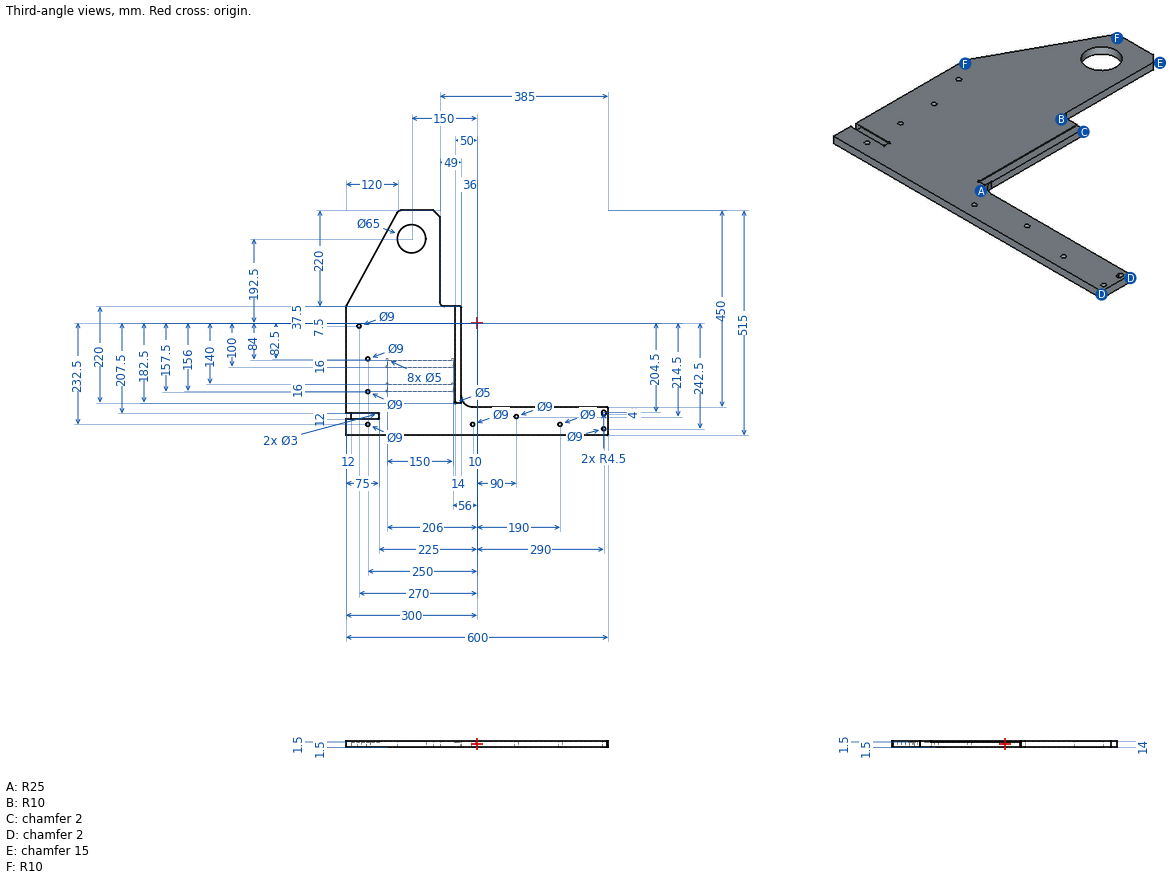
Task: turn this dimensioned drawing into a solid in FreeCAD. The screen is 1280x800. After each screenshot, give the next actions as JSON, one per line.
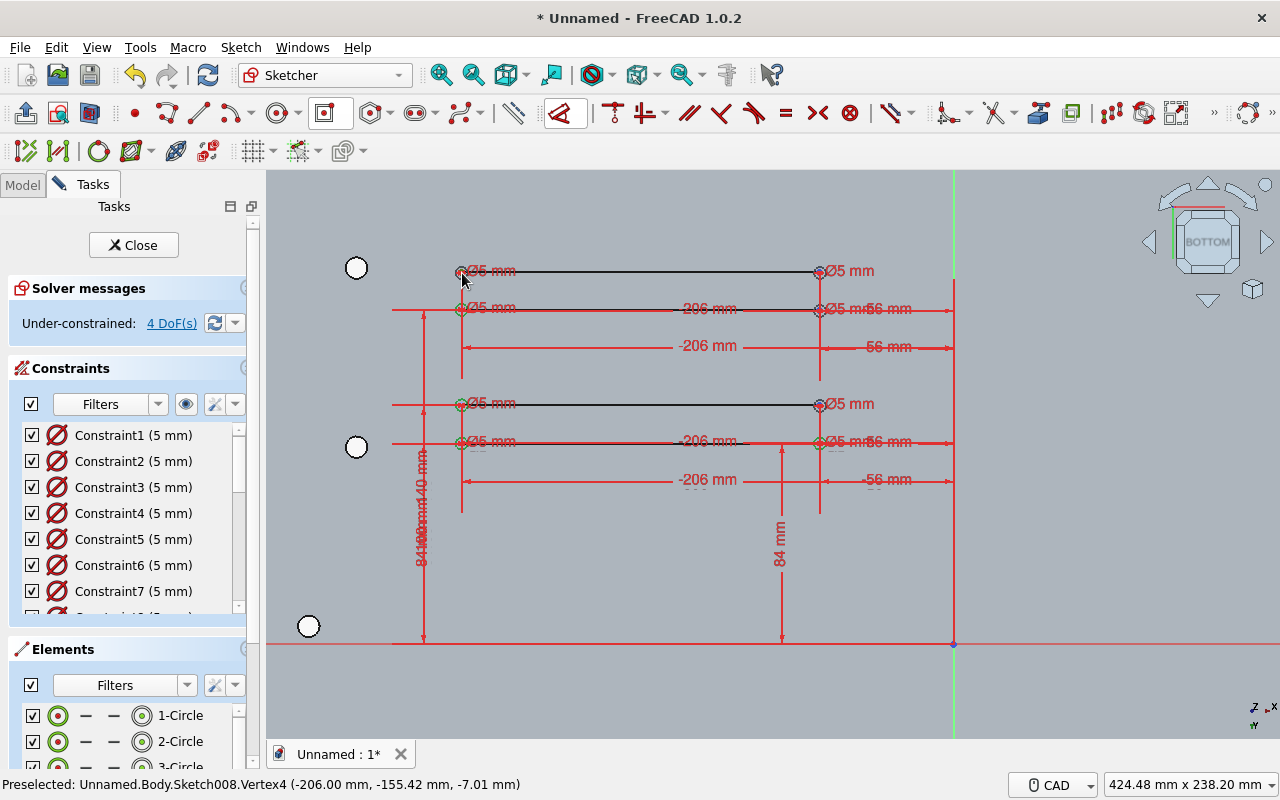
{"action": "left_click", "coordinate": [582, 114]}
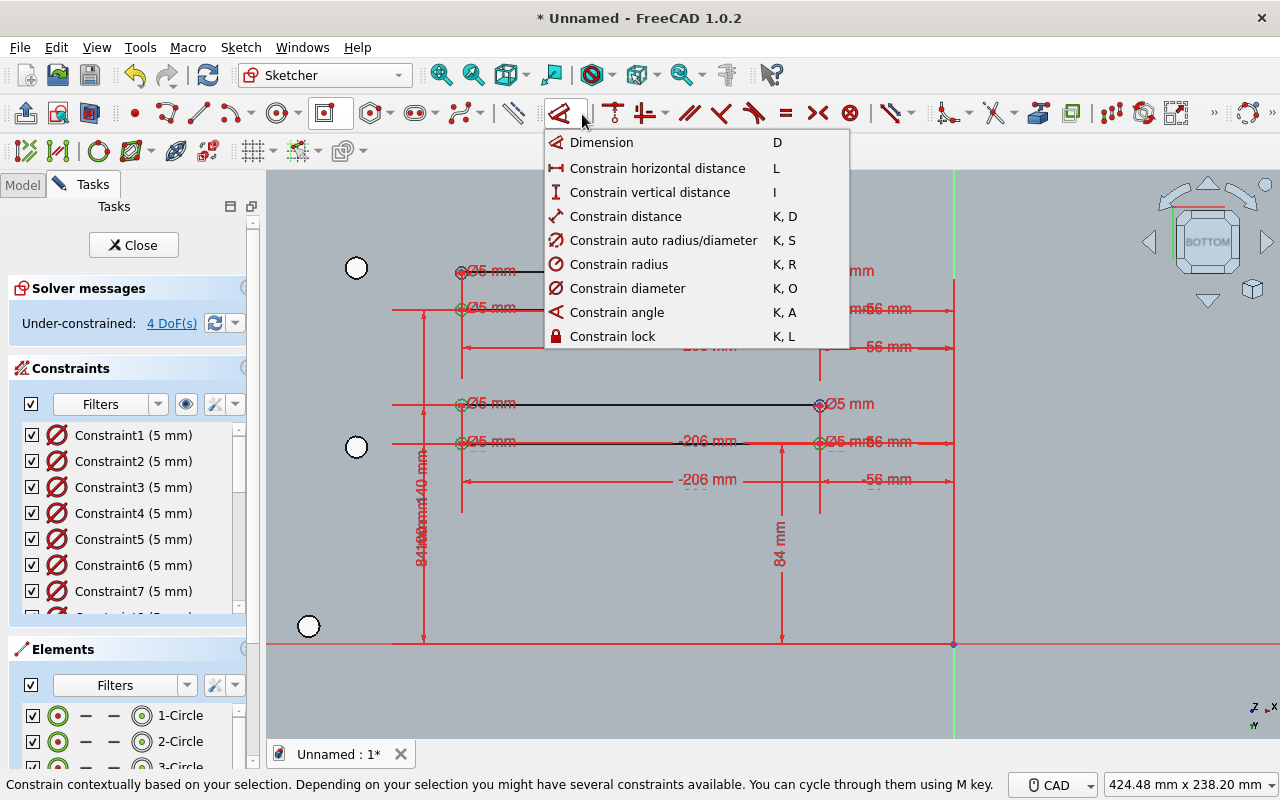
{"action": "left_click", "coordinate": [697, 192]}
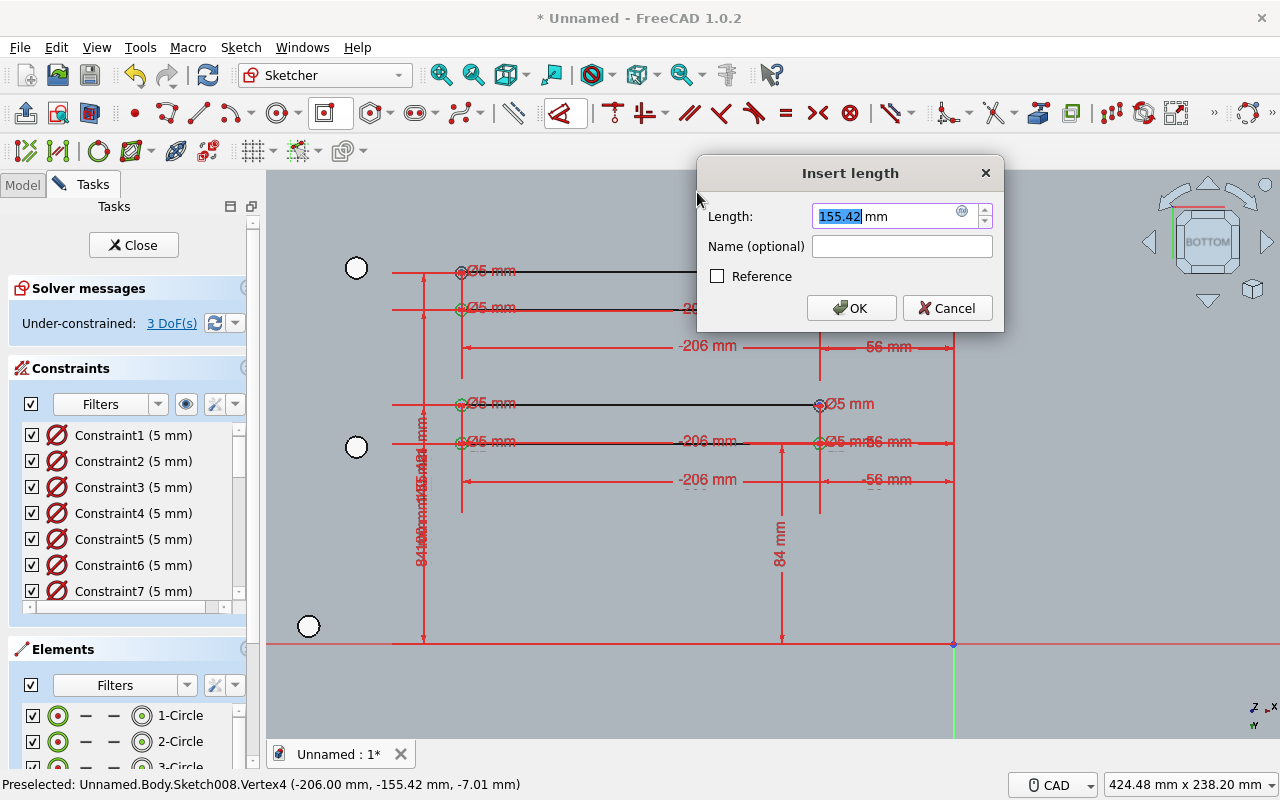
{"action": "type", "text": "156"}
{"action": "key", "text": "Return"}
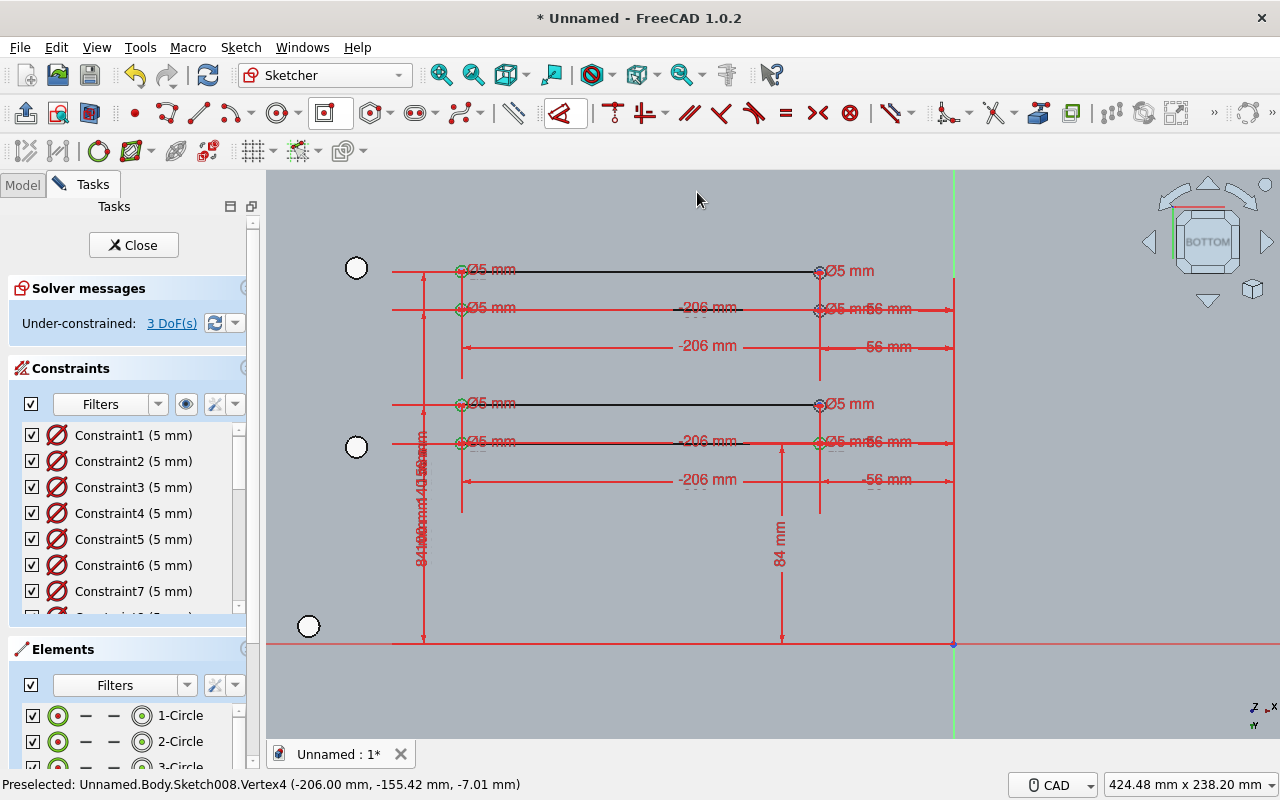
{"action": "left_click", "coordinate": [820, 406]}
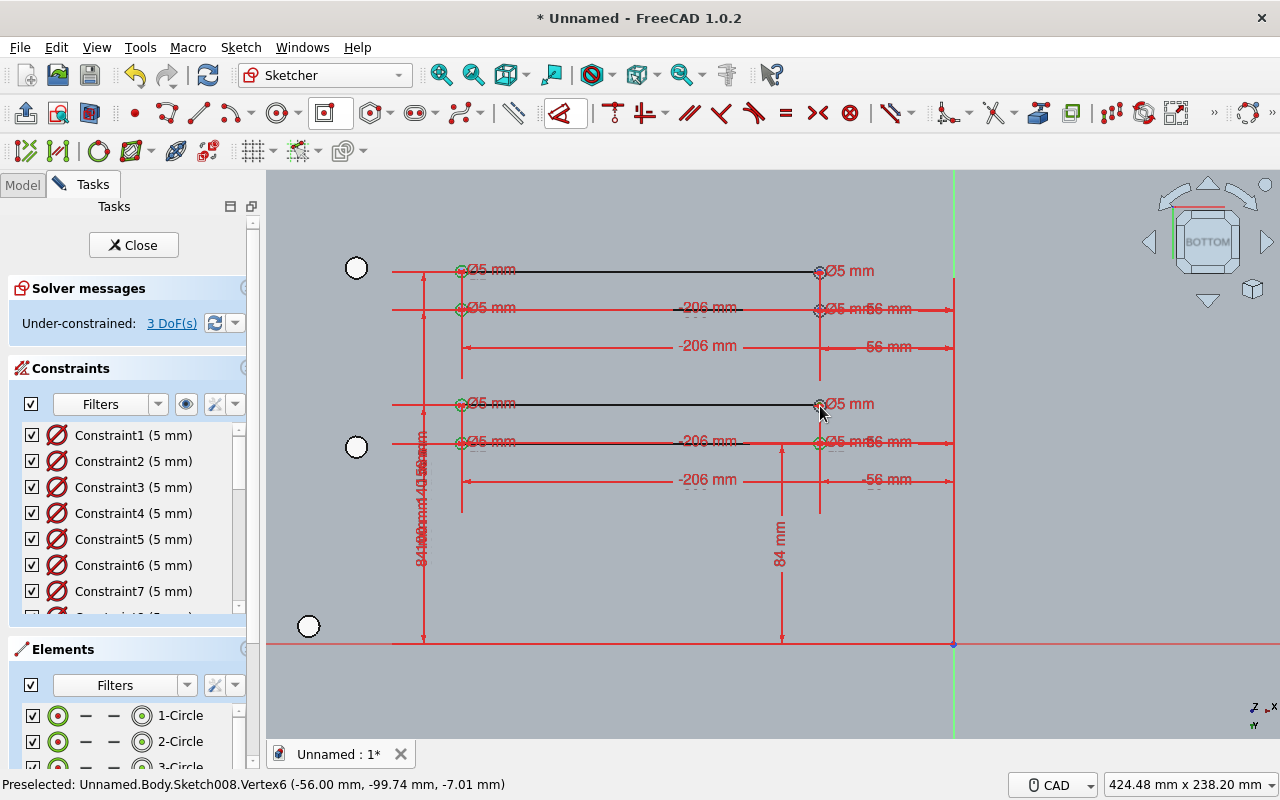
{"action": "key", "text": "i"}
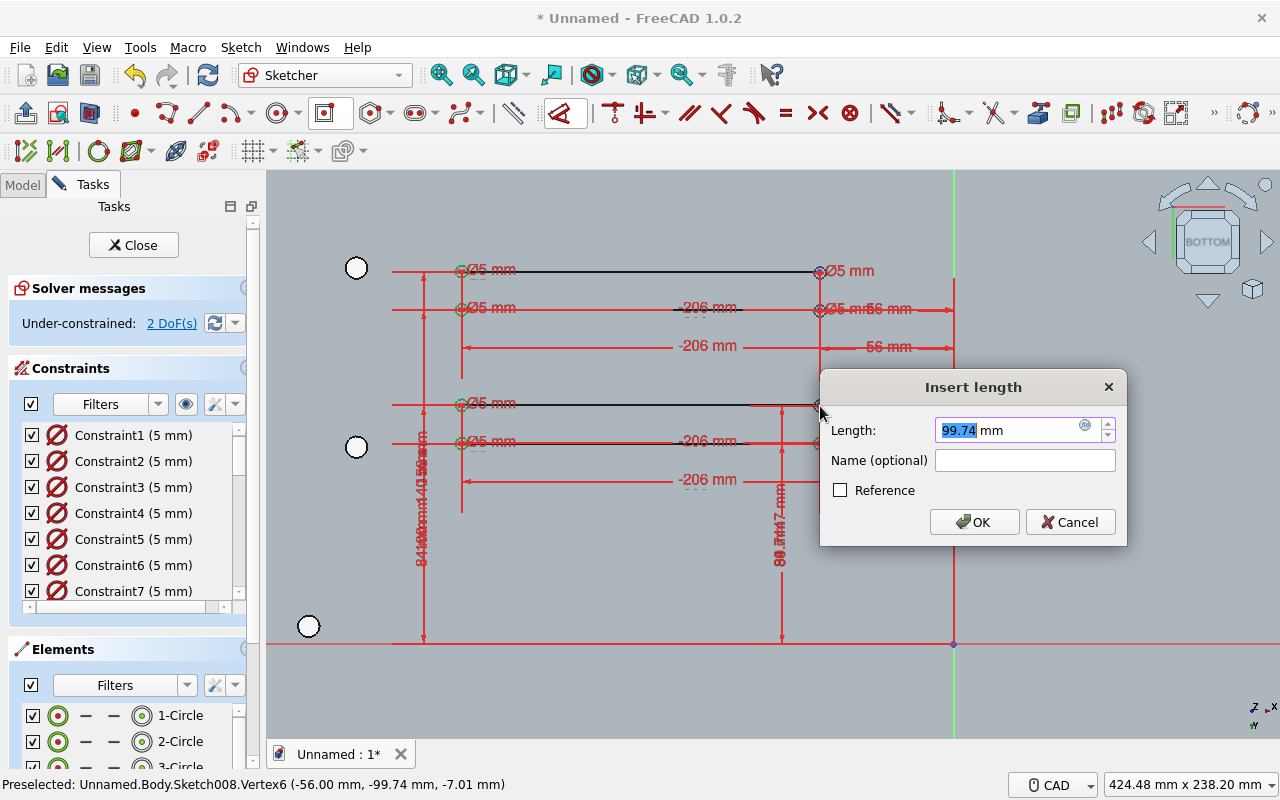
{"action": "type", "text": "100"}
{"action": "key", "text": "Return"}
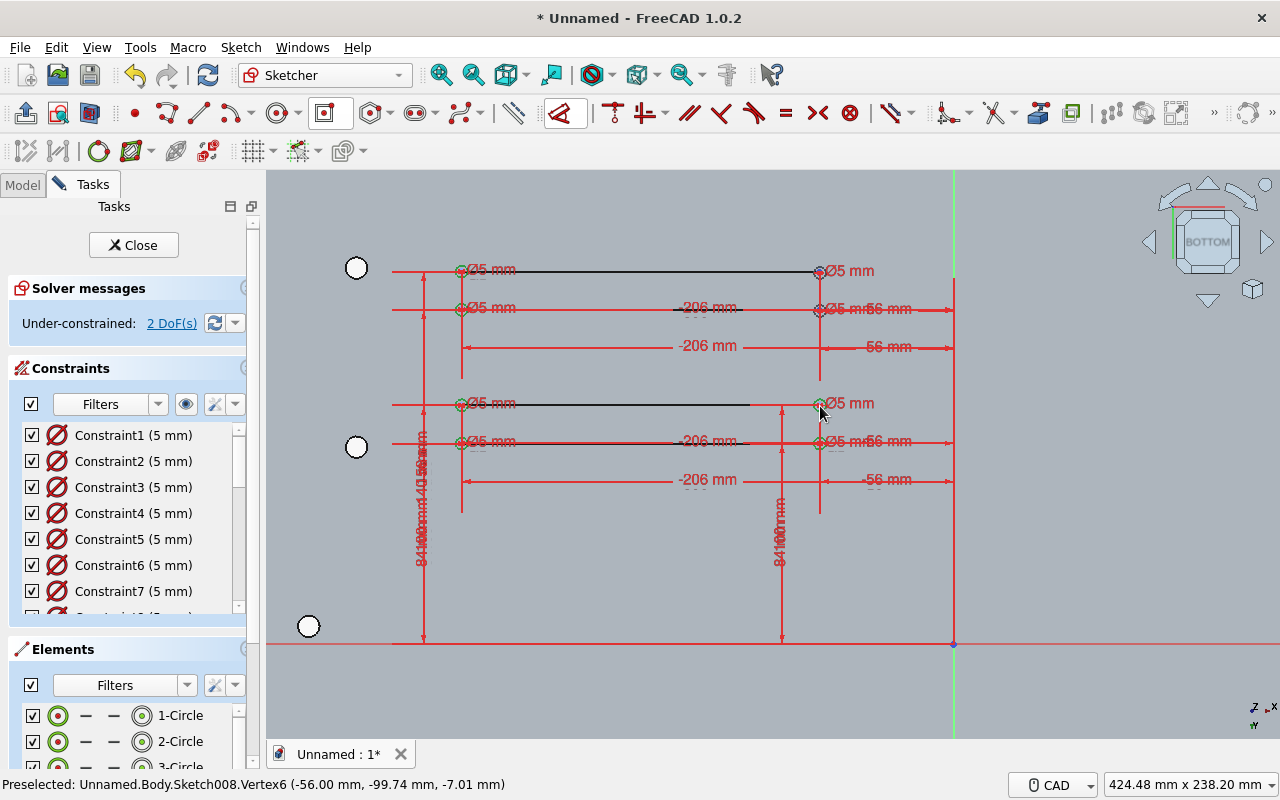
{"action": "left_click", "coordinate": [820, 311]}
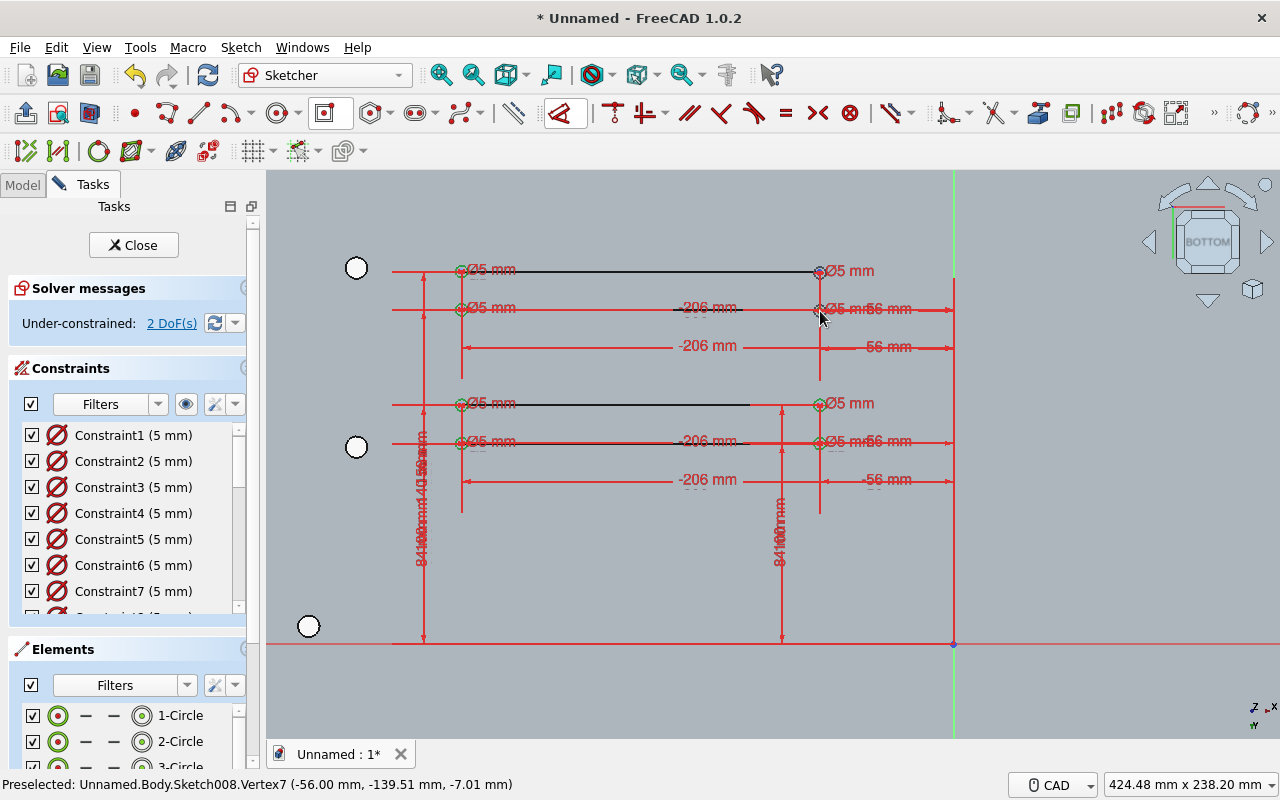
{"action": "left_click", "coordinate": [582, 114]}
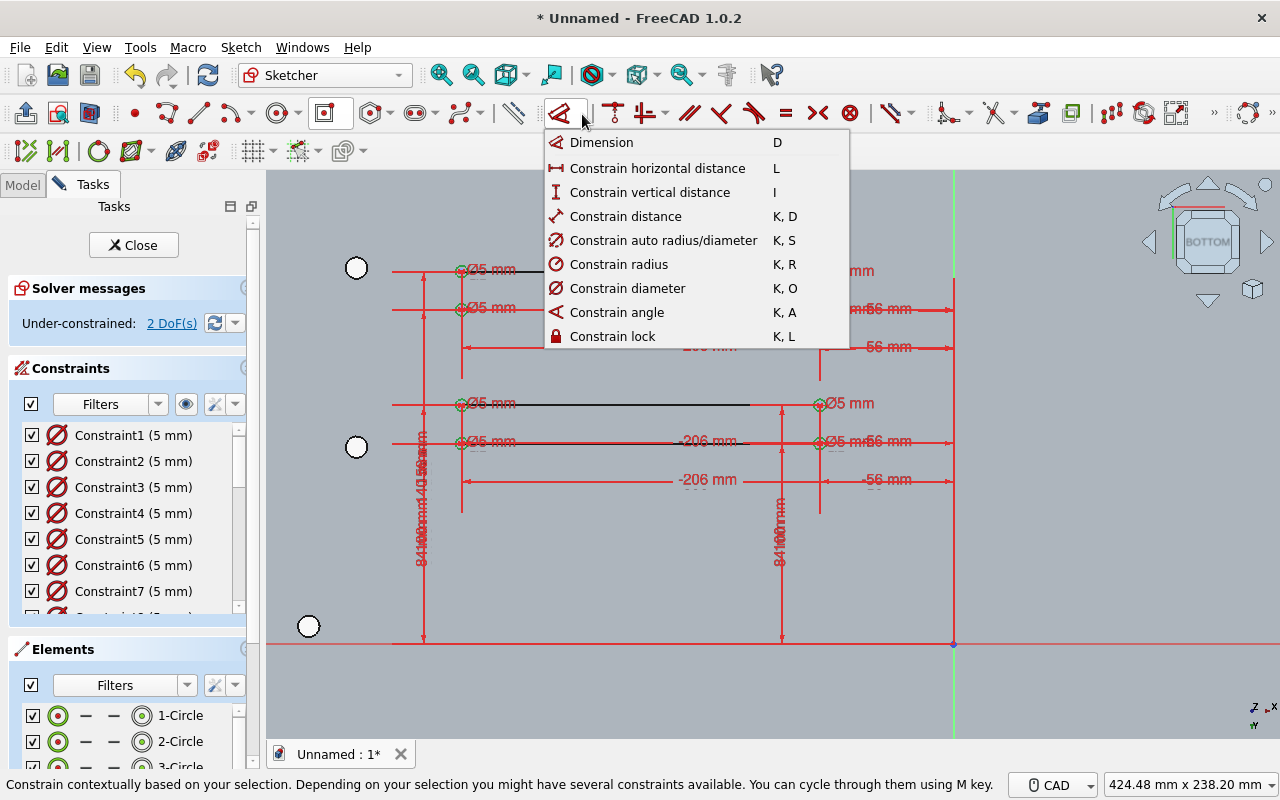
{"action": "left_click", "coordinate": [697, 192]}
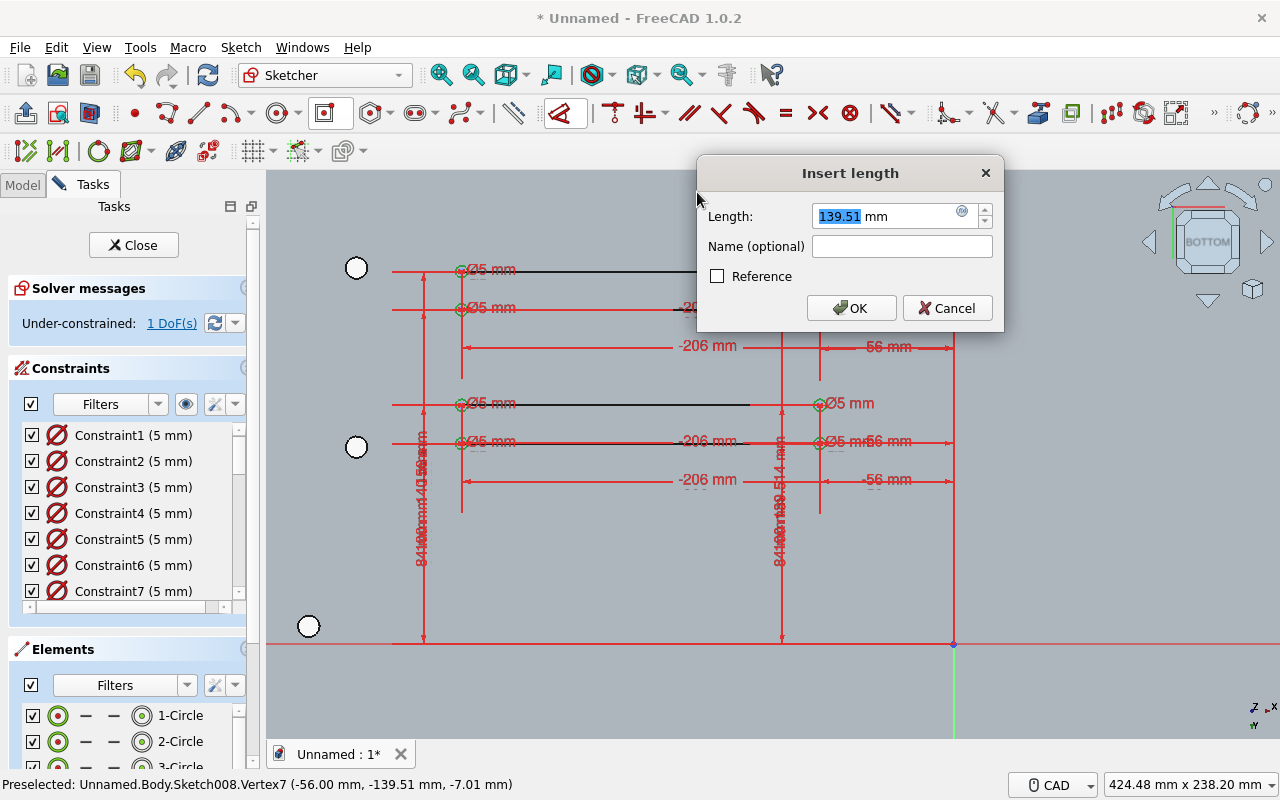
{"action": "type", "text": "140"}
{"action": "key", "text": "Return"}